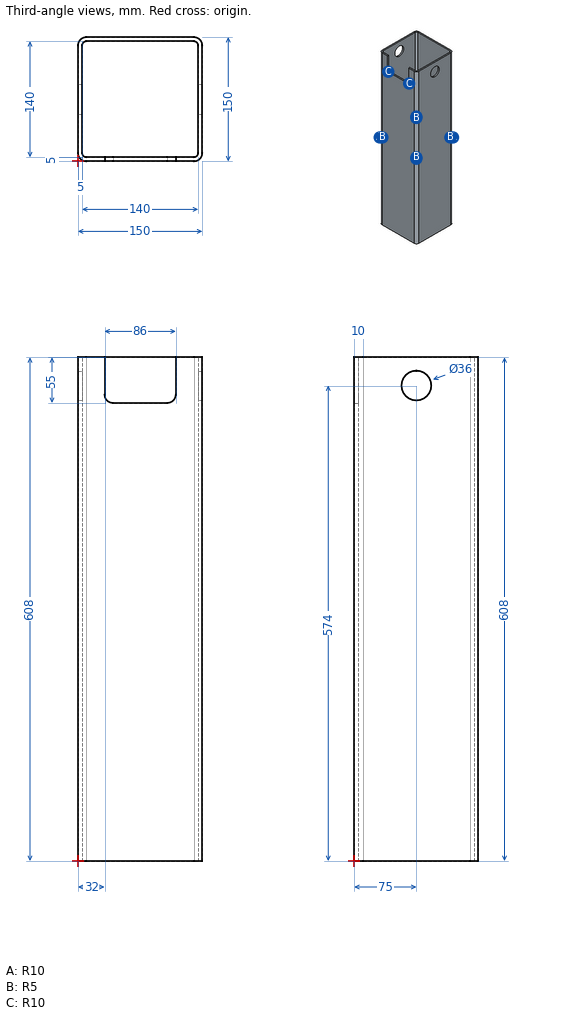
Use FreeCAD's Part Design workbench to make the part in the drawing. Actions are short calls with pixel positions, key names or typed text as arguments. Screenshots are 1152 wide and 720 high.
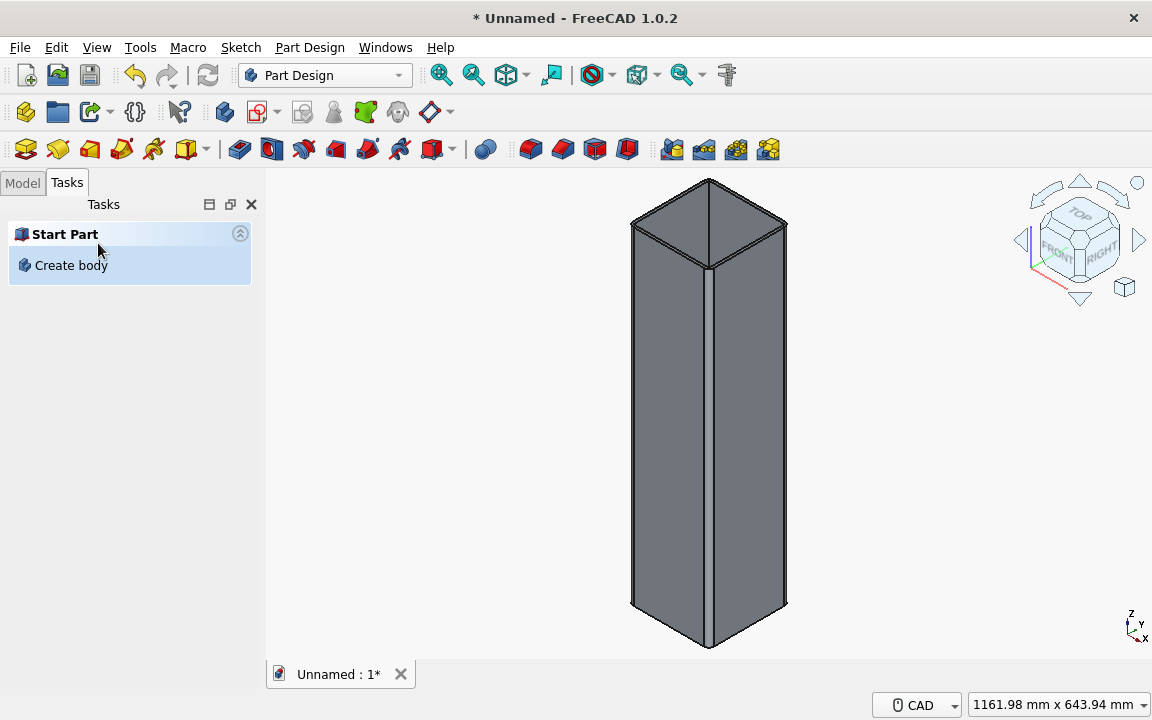
key(2)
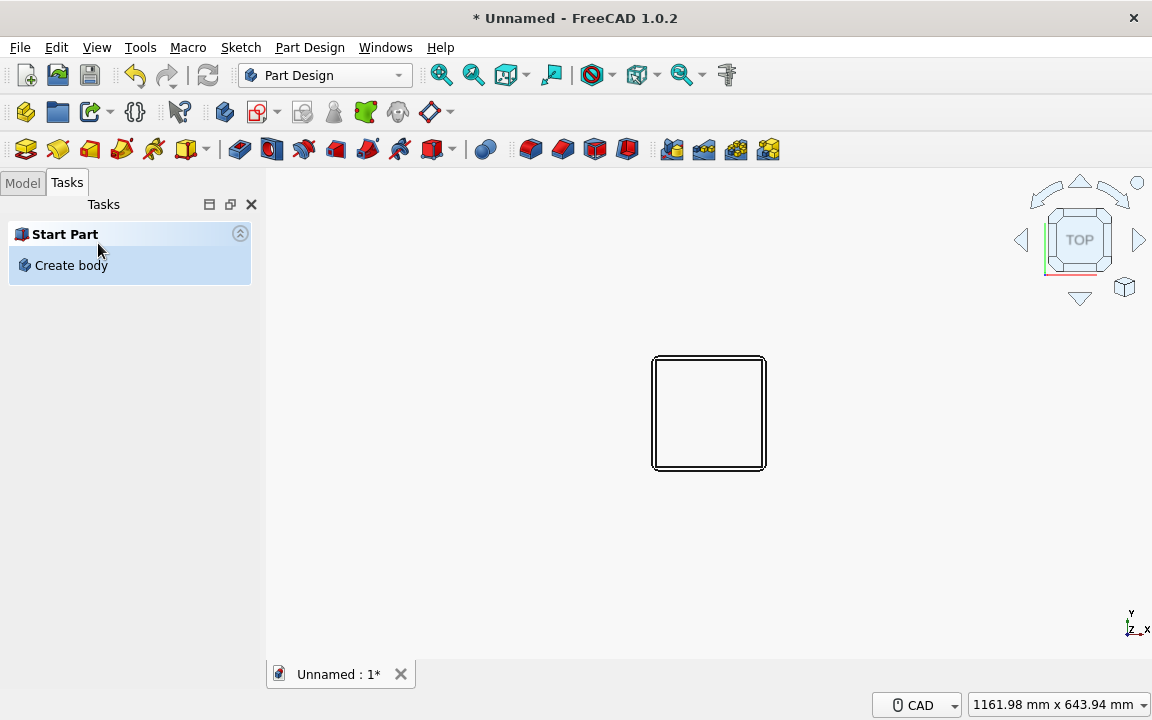
key(v)
key(f)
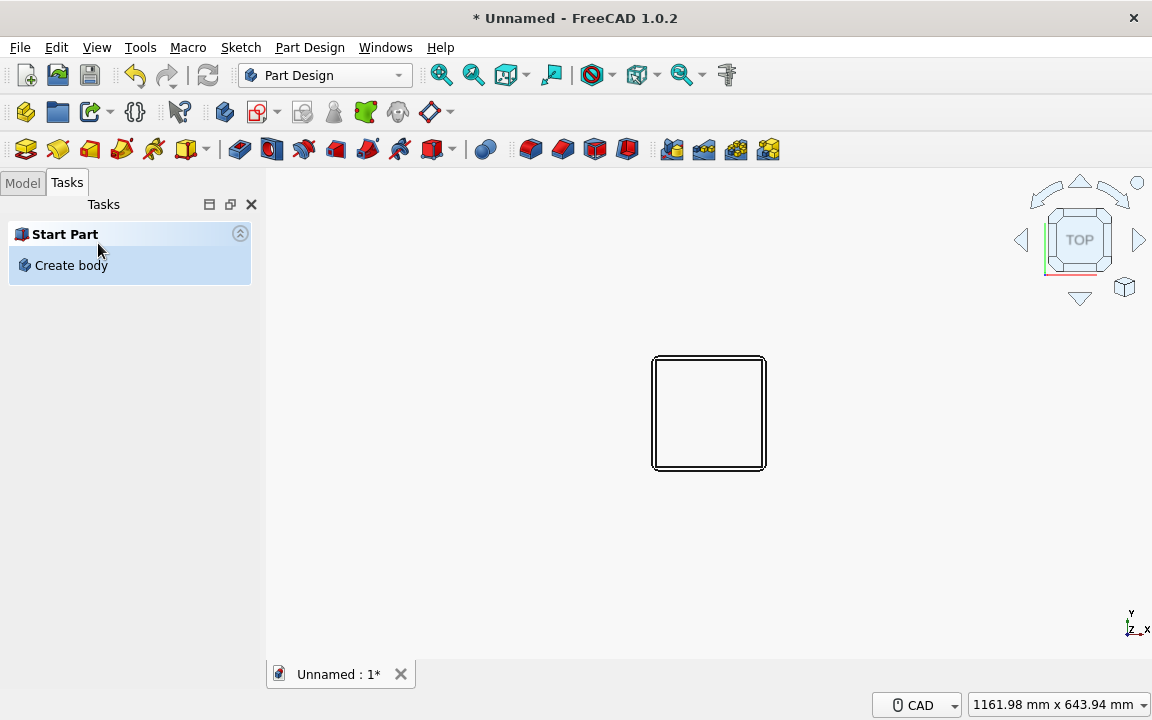
key(0)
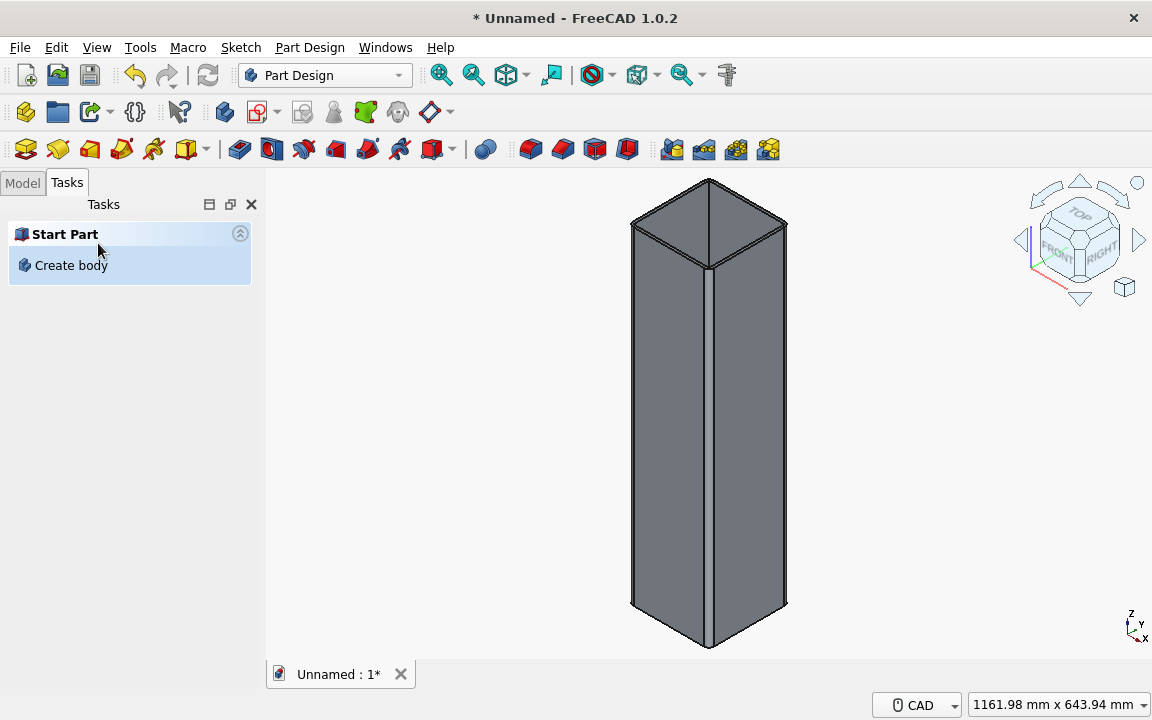
key(1)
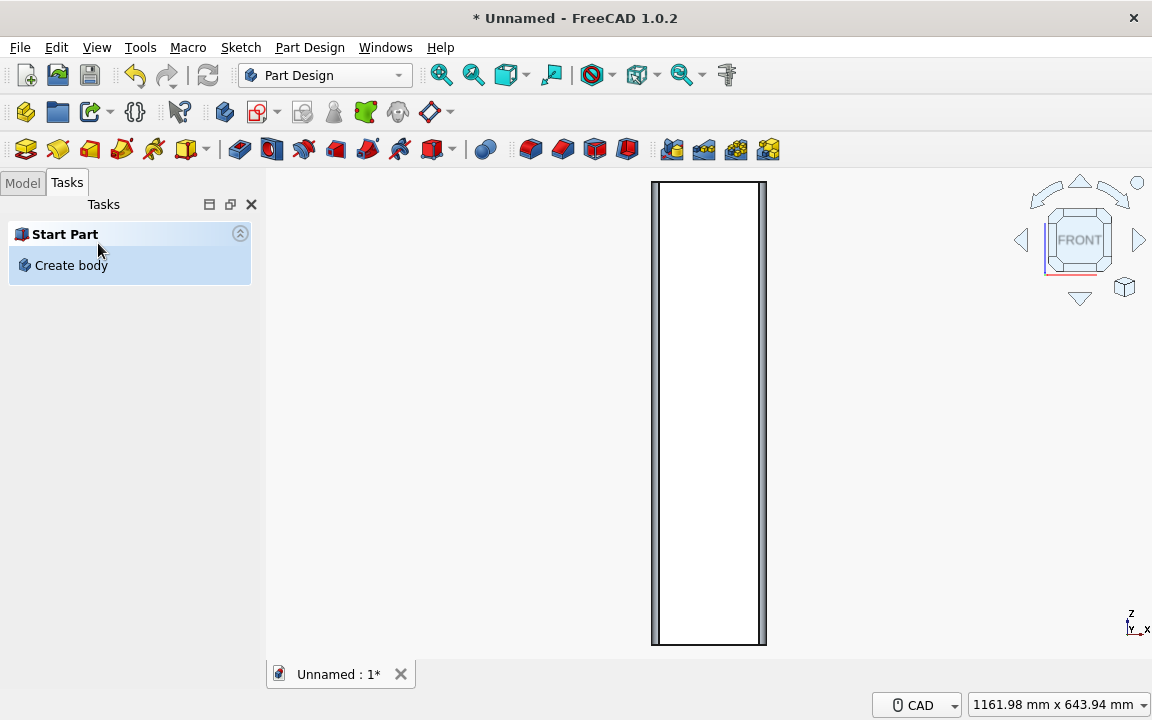
key(3)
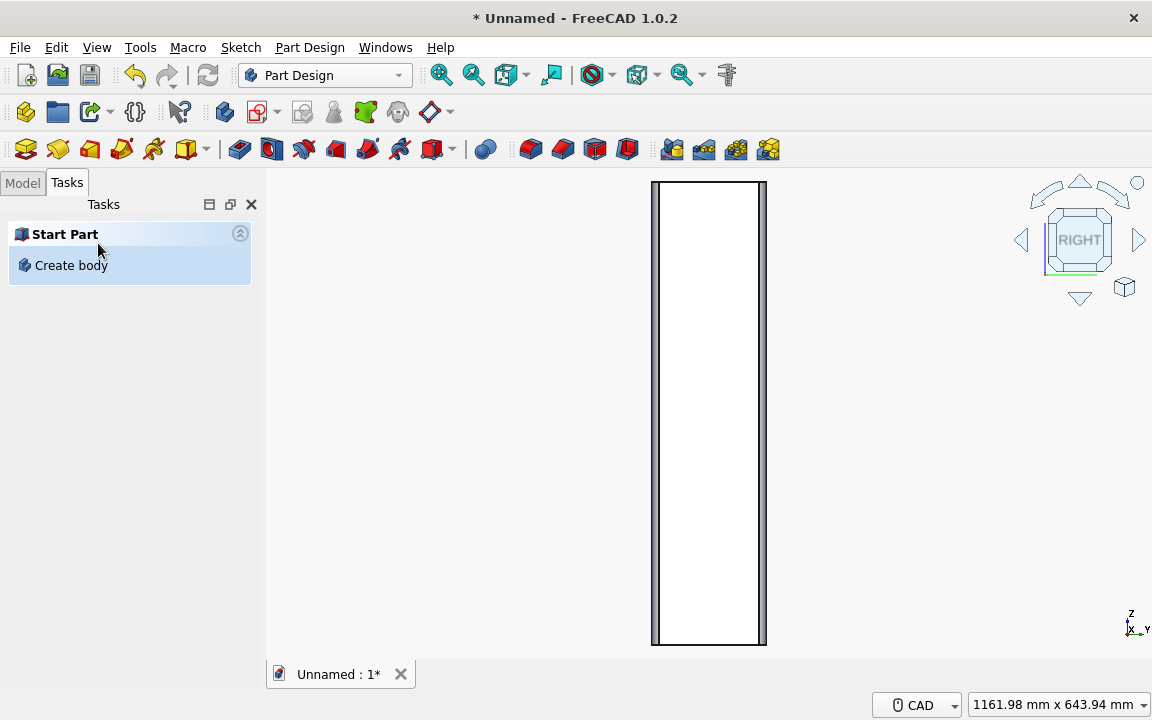
key(5)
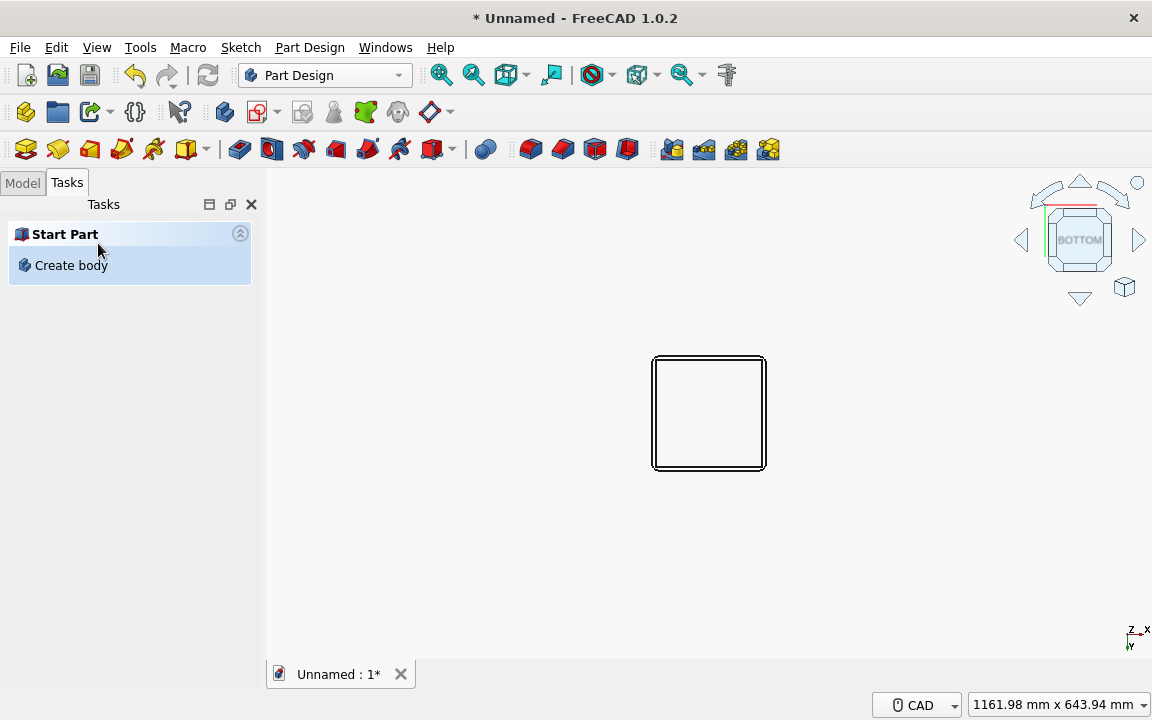
click(442, 76)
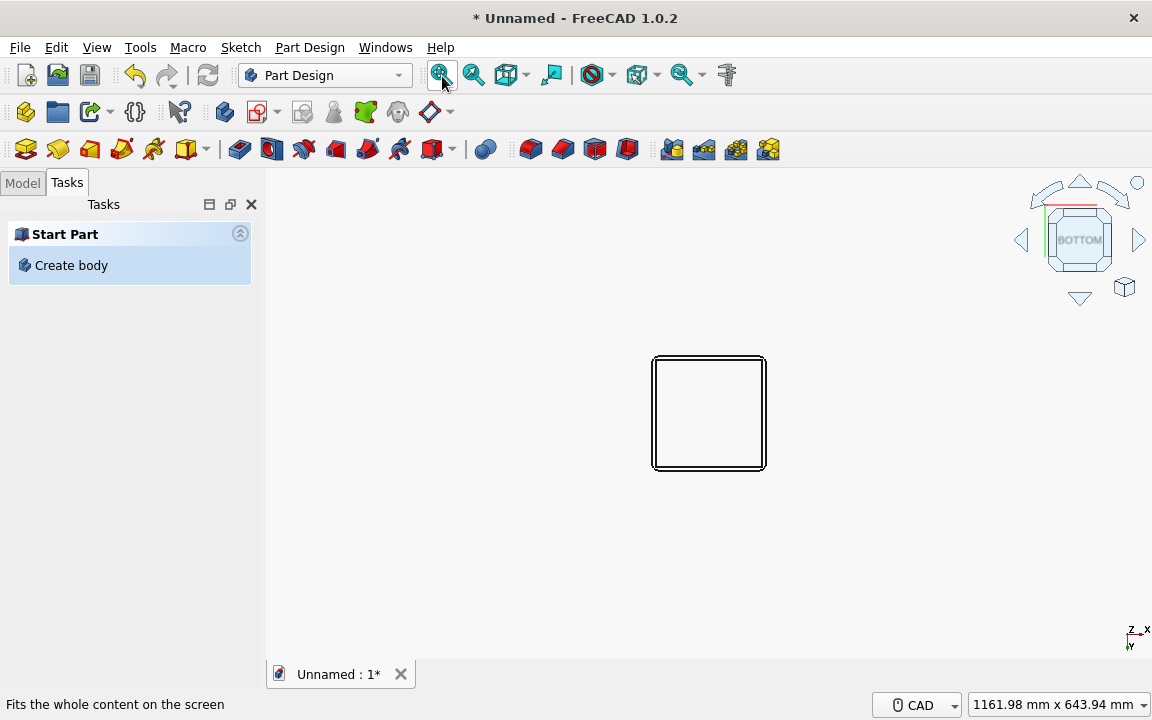
key(4)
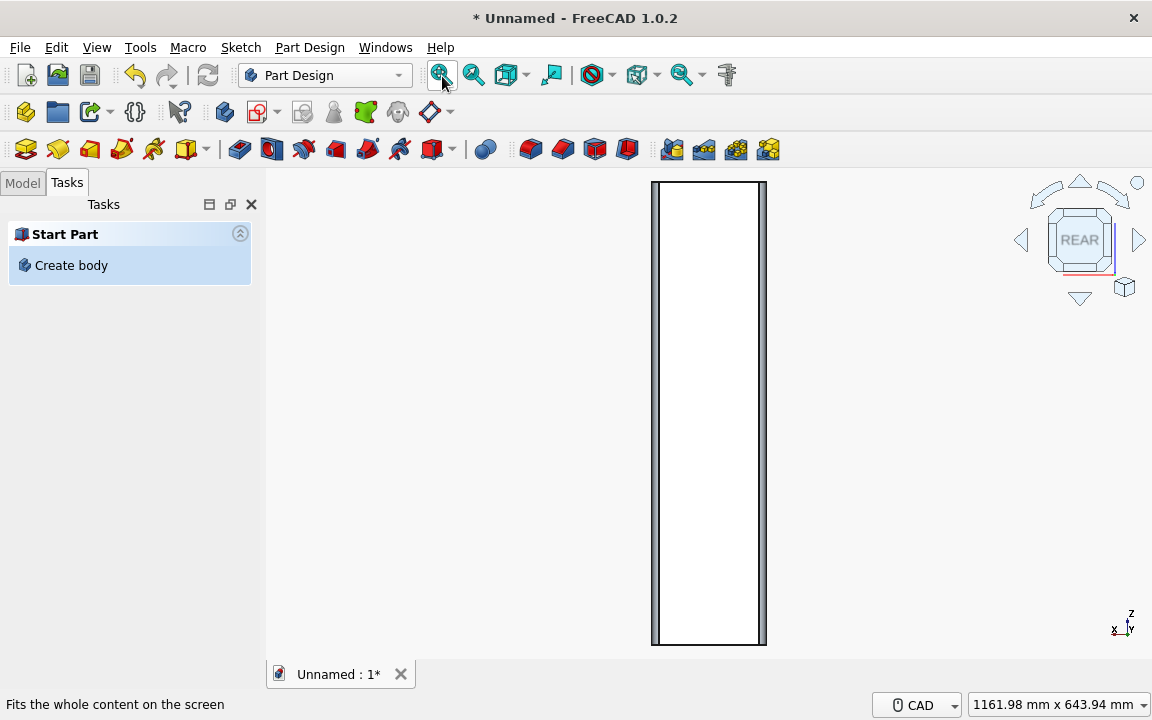
key(6)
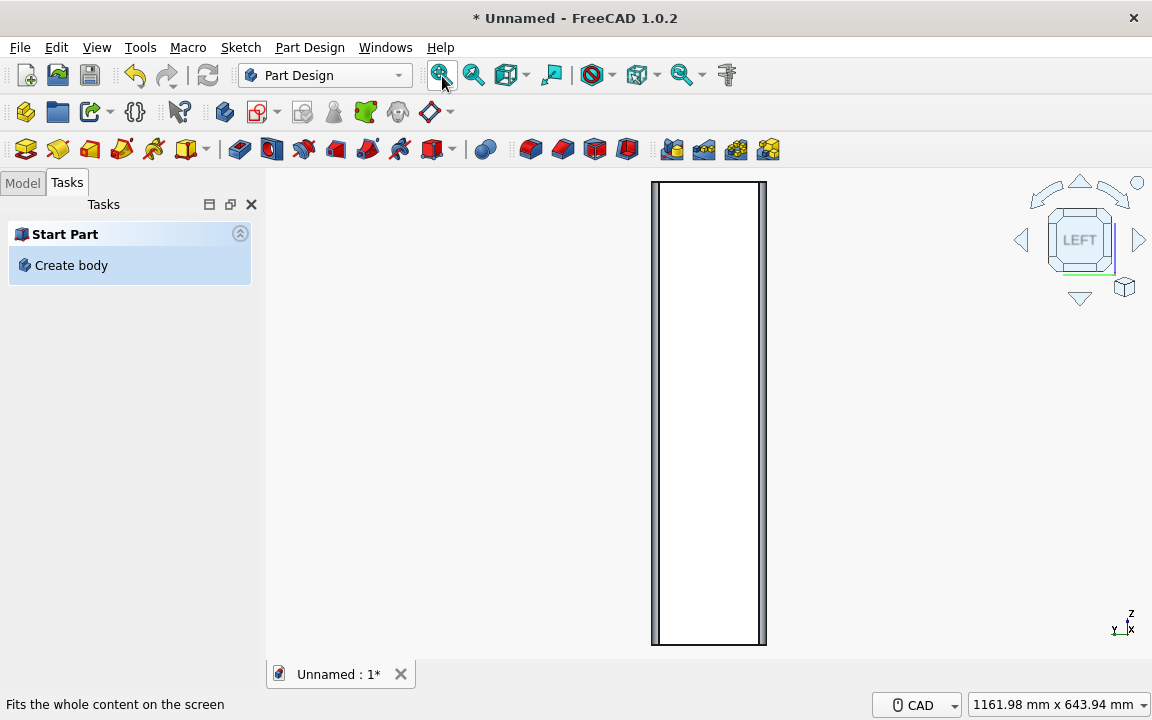
key(v)
key(3)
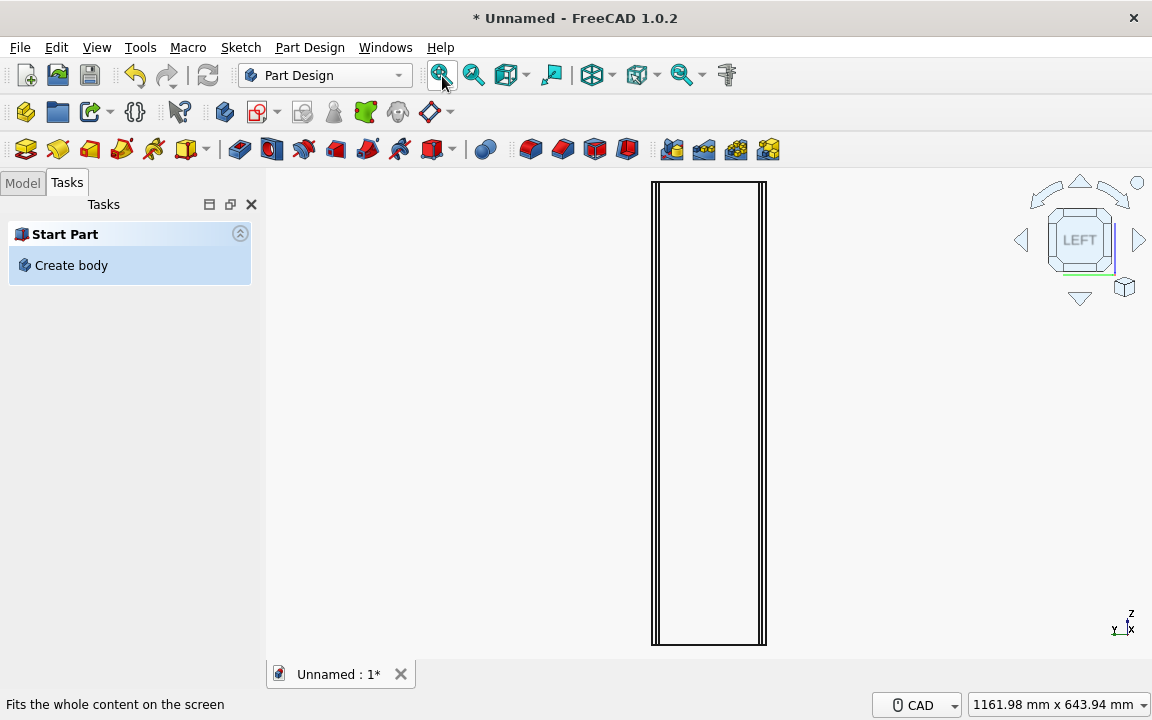
key(0)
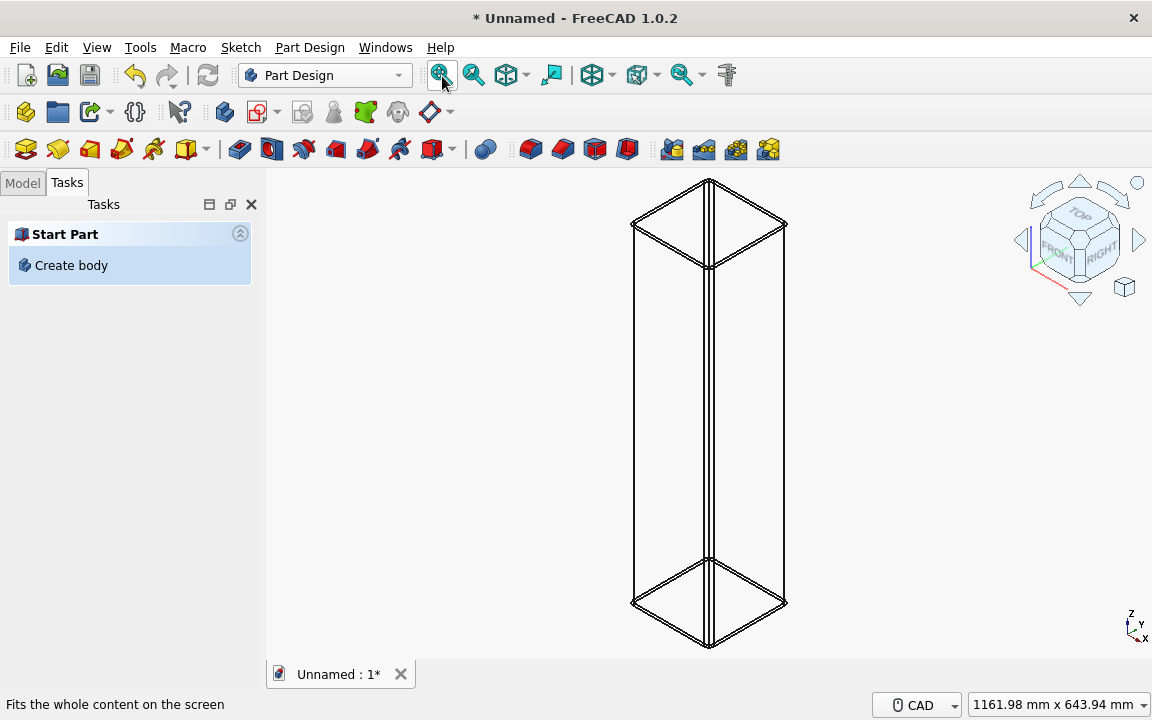
scroll(709, 369, up, 6)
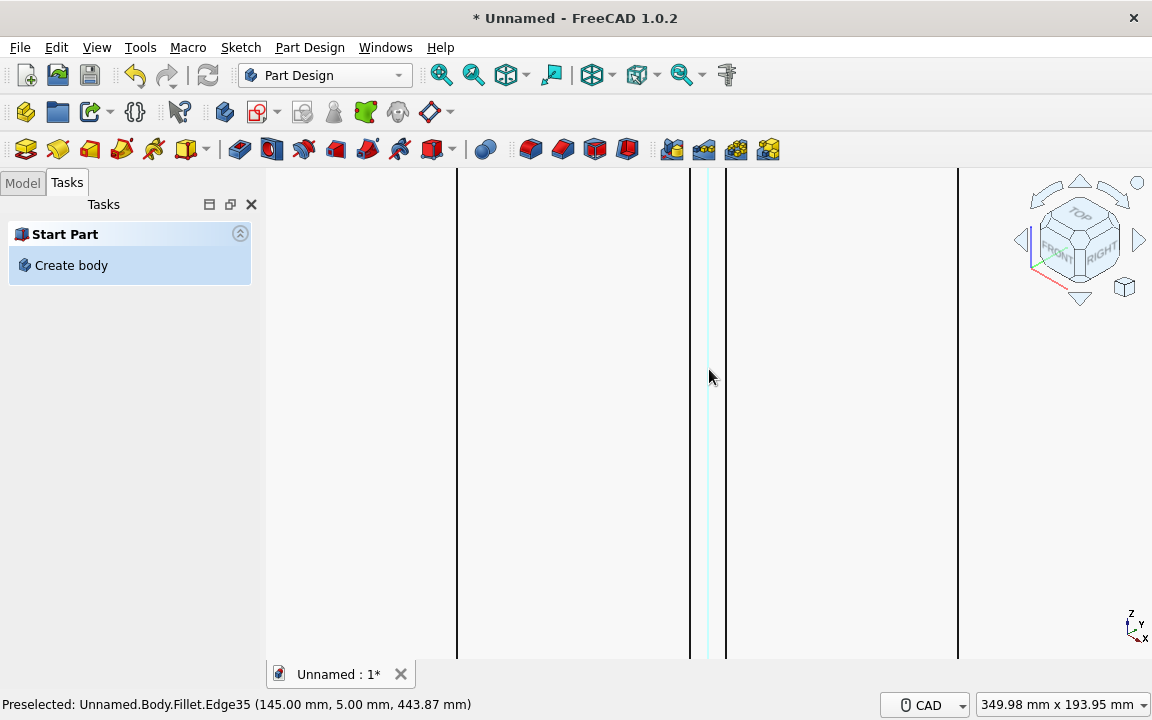
click(708, 534)